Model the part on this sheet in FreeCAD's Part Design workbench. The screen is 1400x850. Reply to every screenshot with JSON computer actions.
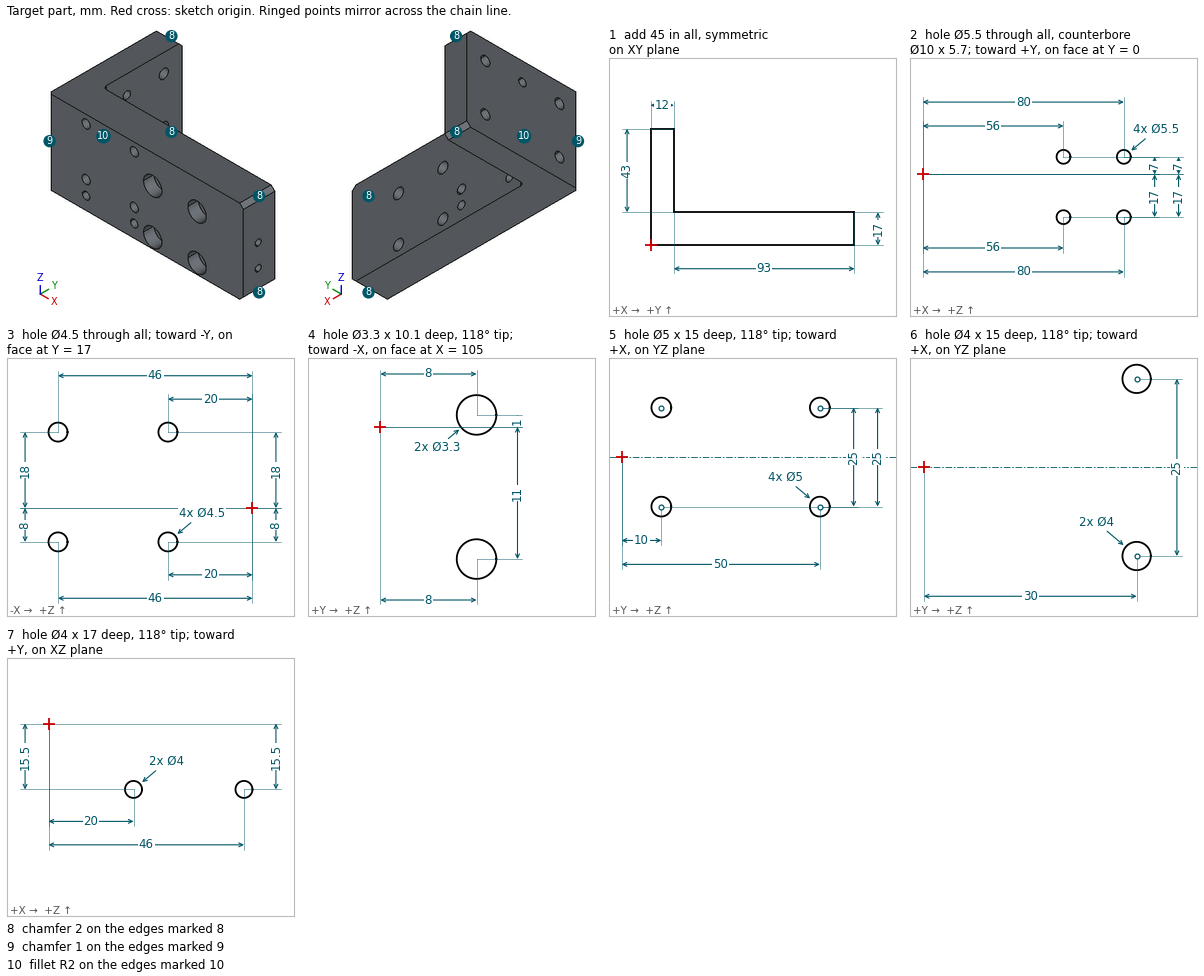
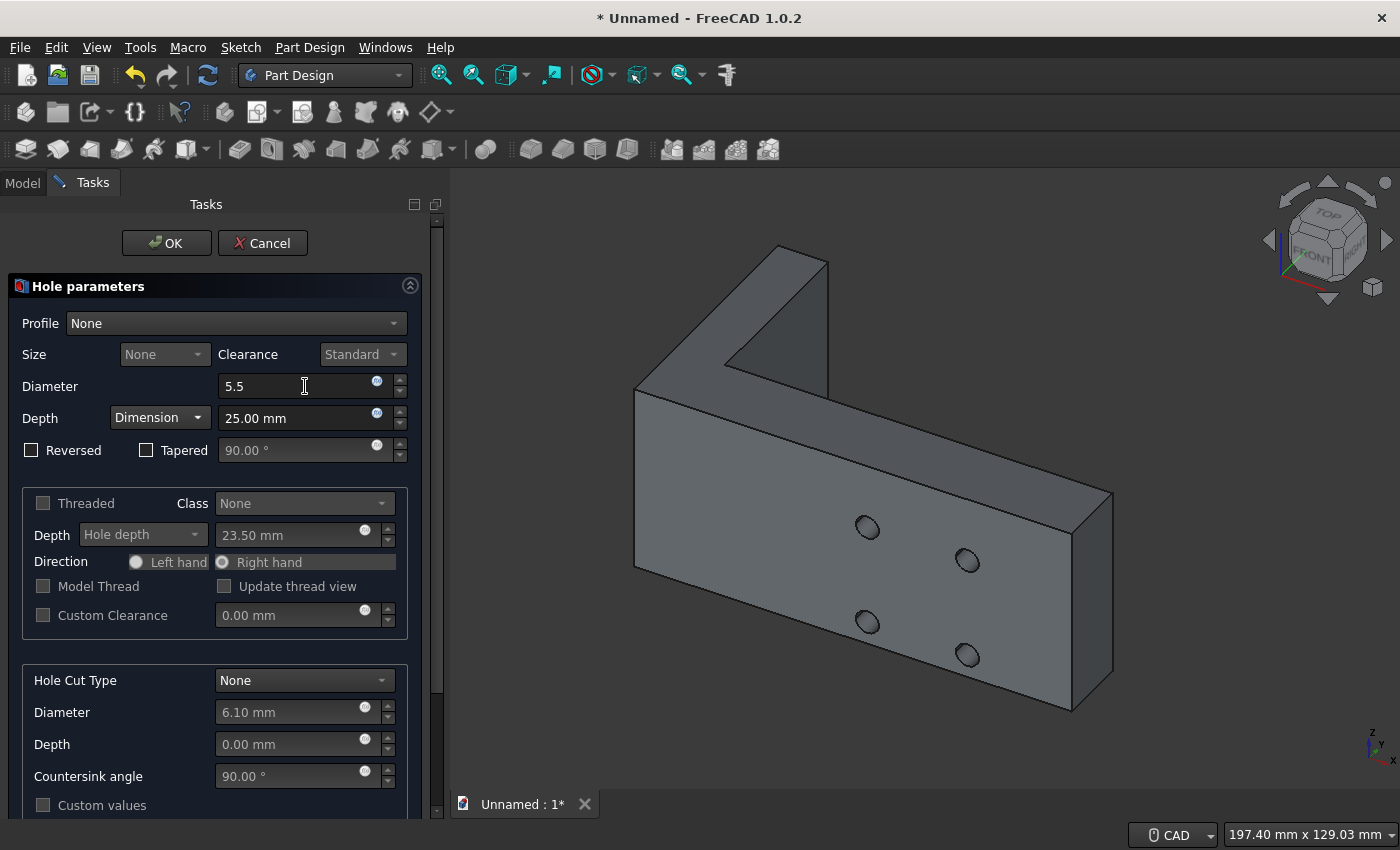
{"action": "left_click", "coordinate": [161, 418]}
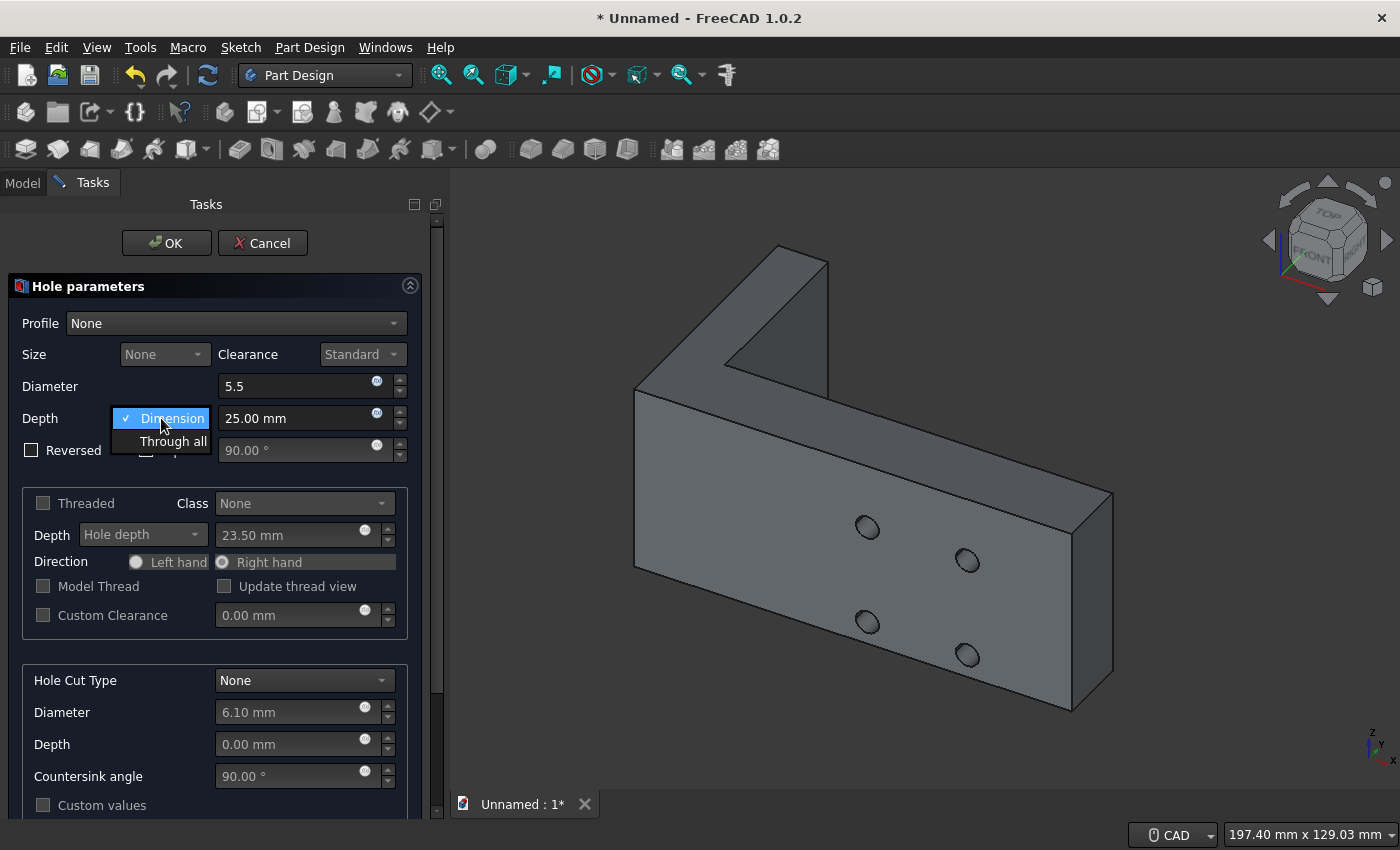
{"action": "left_click", "coordinate": [160, 442]}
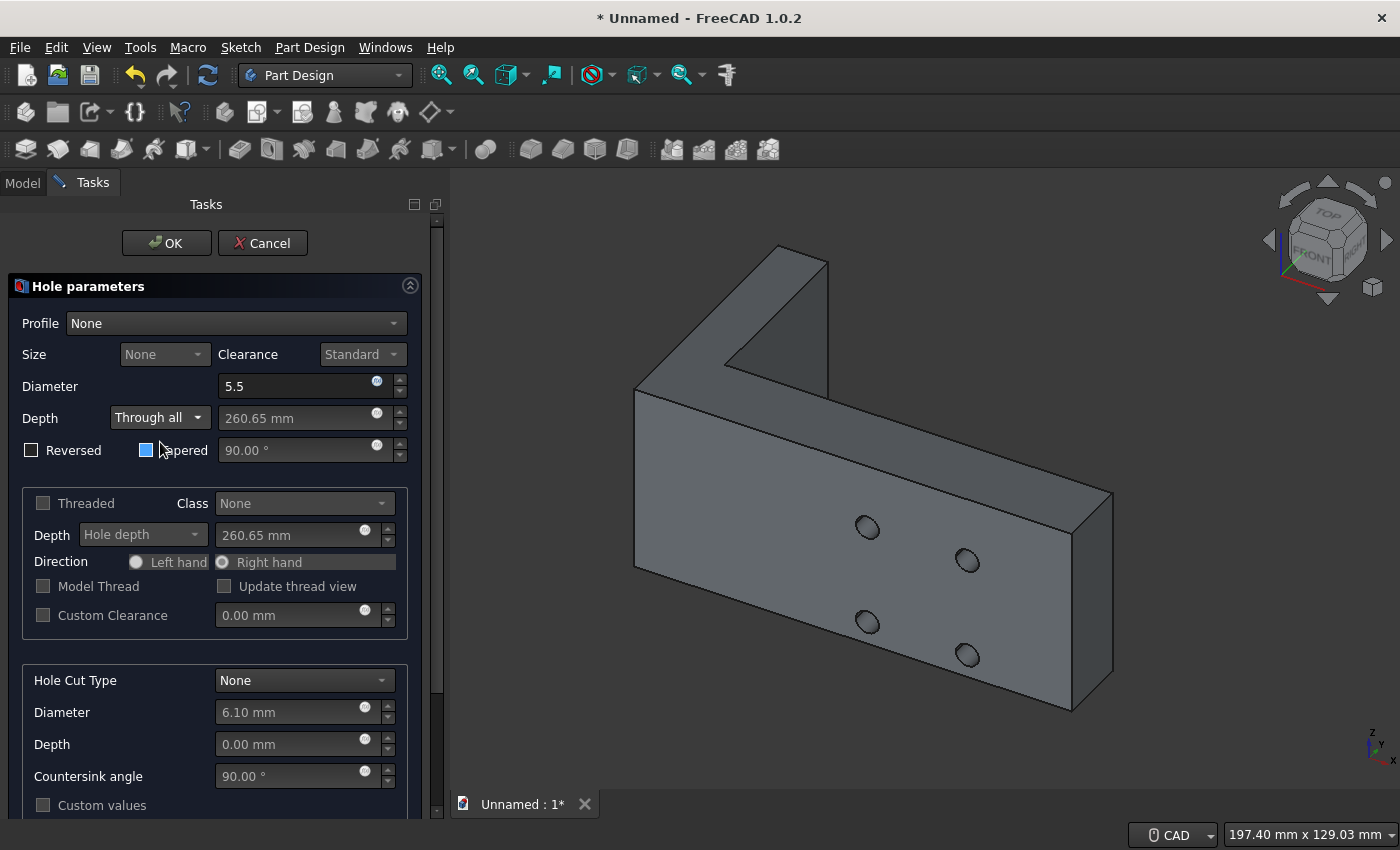
{"action": "left_click", "coordinate": [306, 680]}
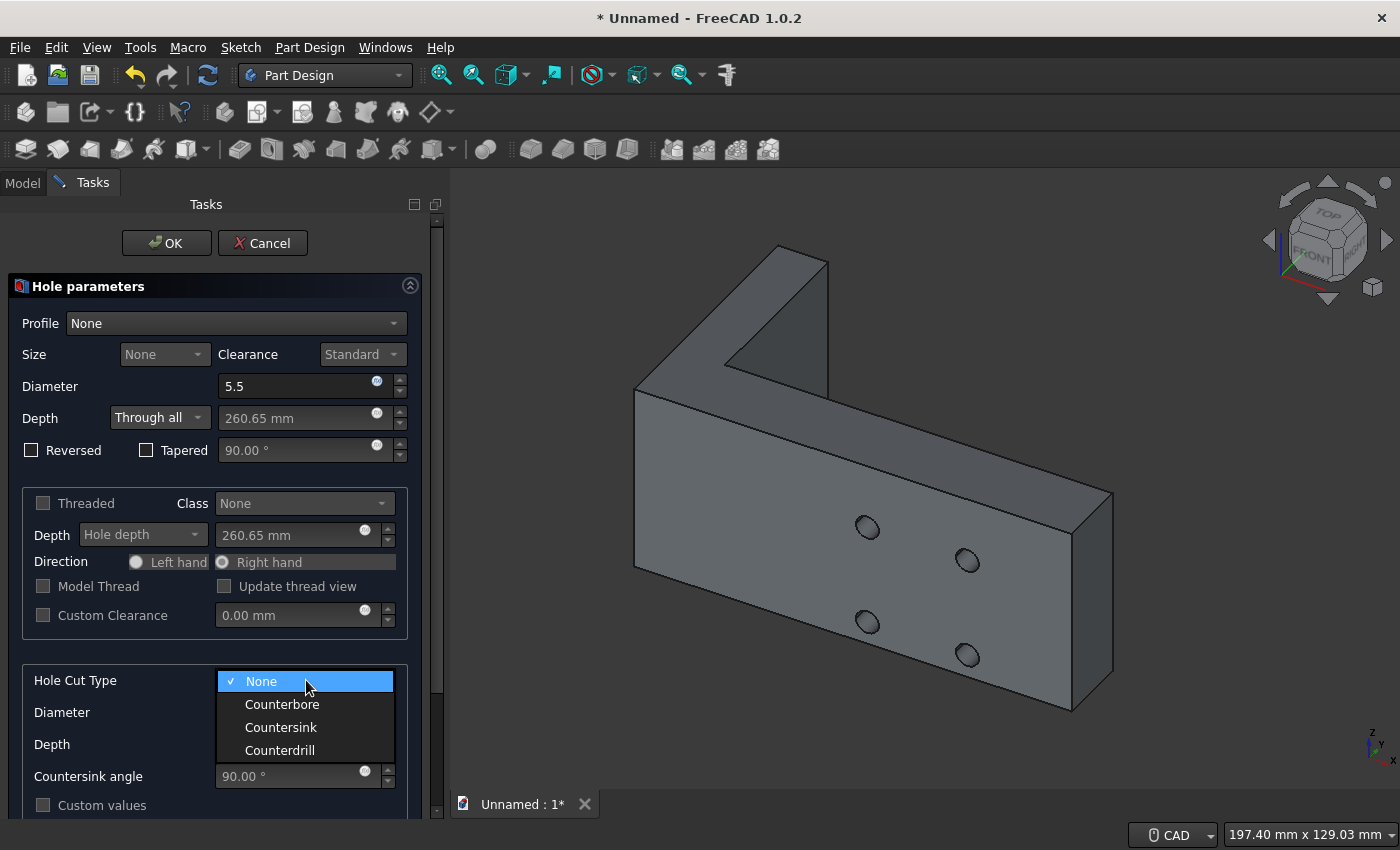
{"action": "left_click", "coordinate": [304, 704]}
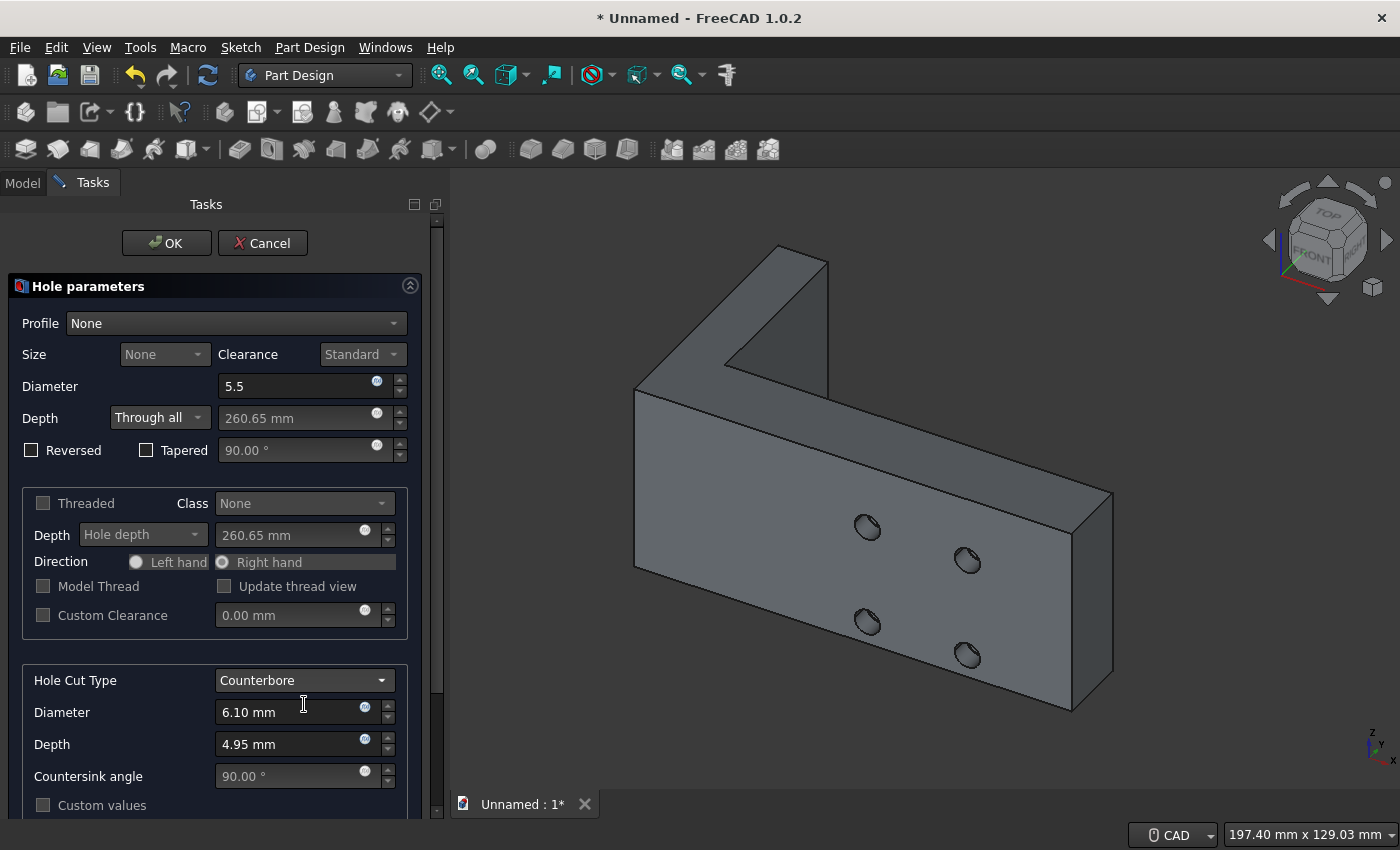
{"action": "triple_click", "coordinate": [298, 712]}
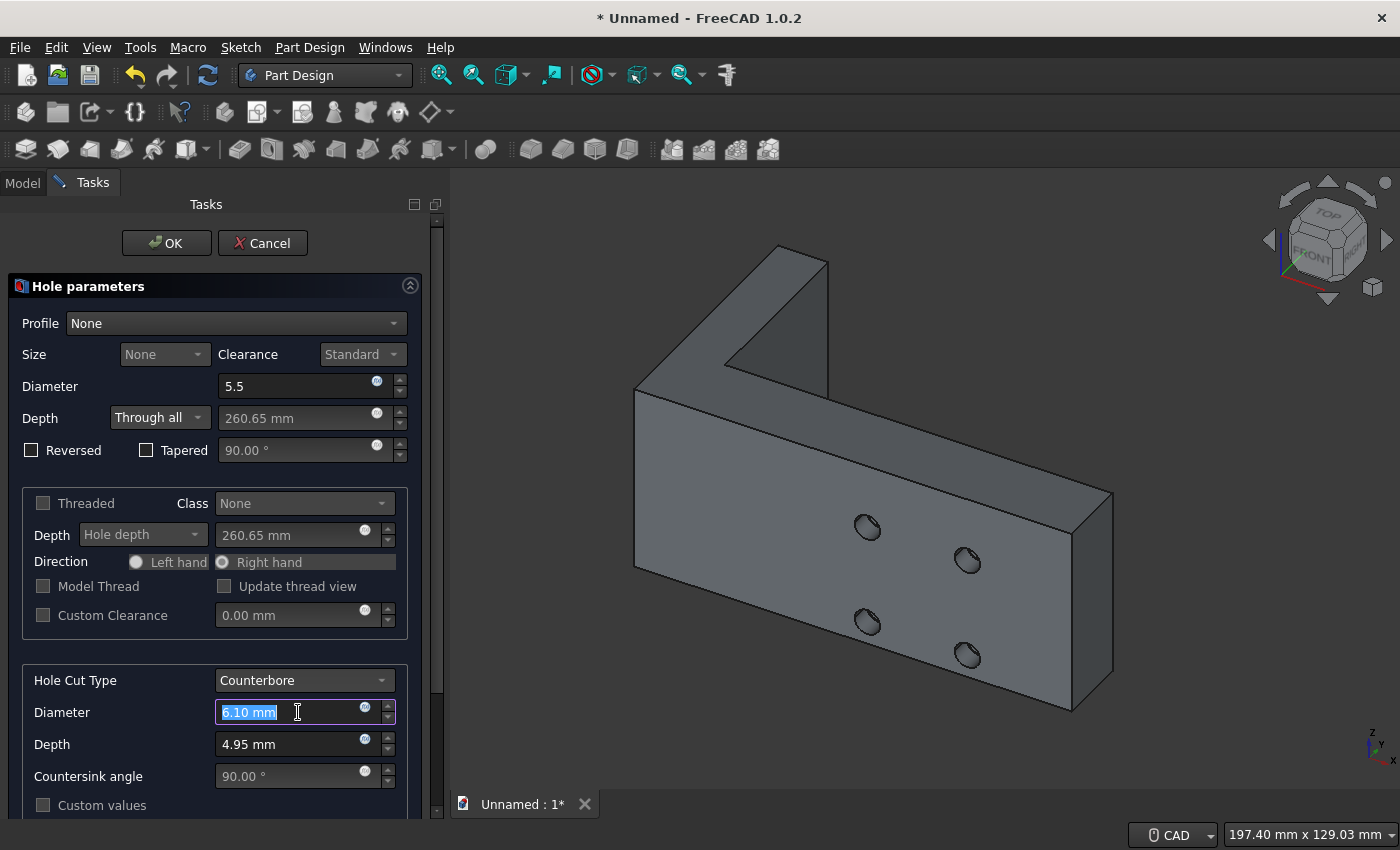
{"action": "type", "text": "10"}
{"action": "key", "text": "Tab"}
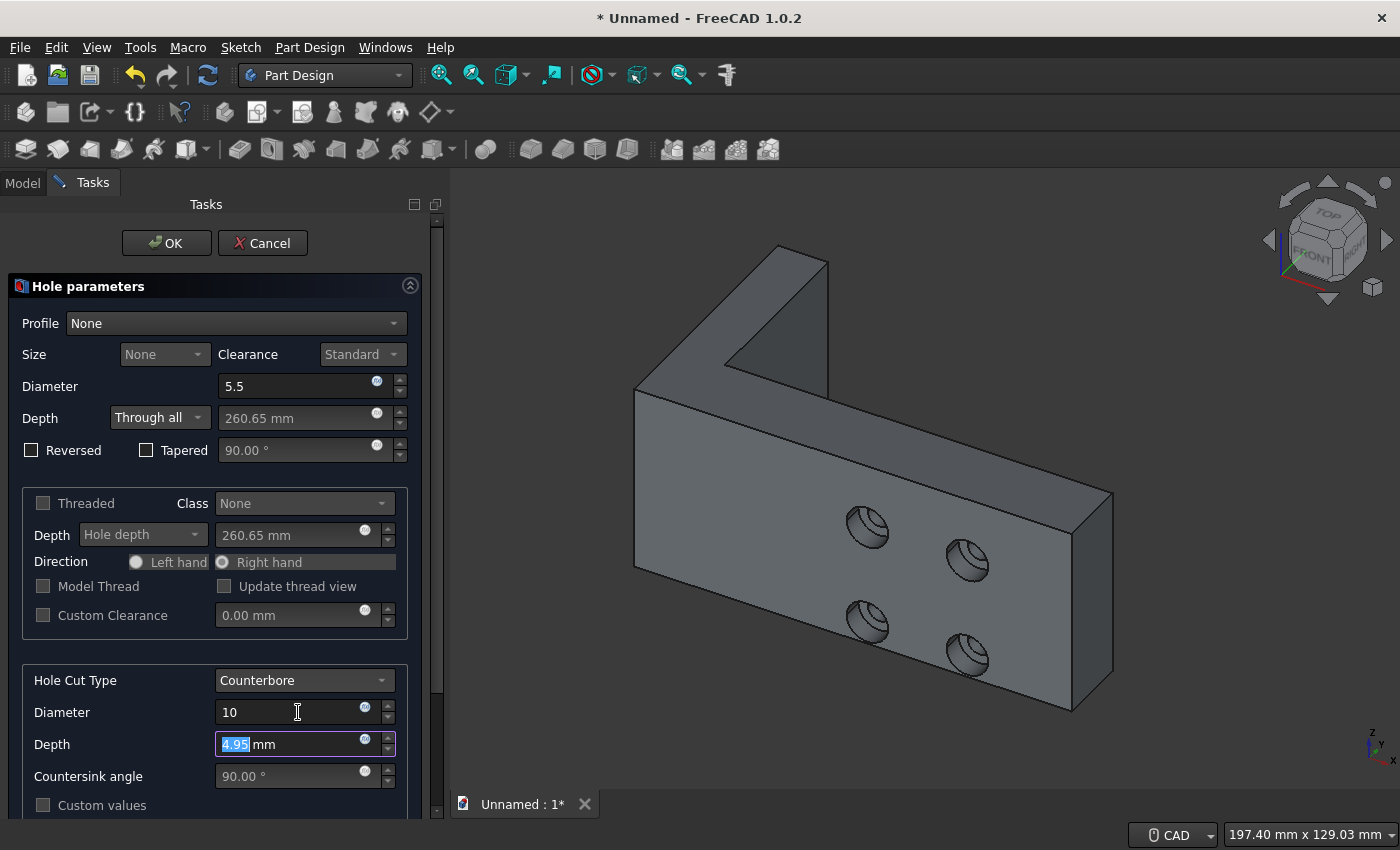
{"action": "type", "text": "5.7"}
{"action": "key", "text": "Tab"}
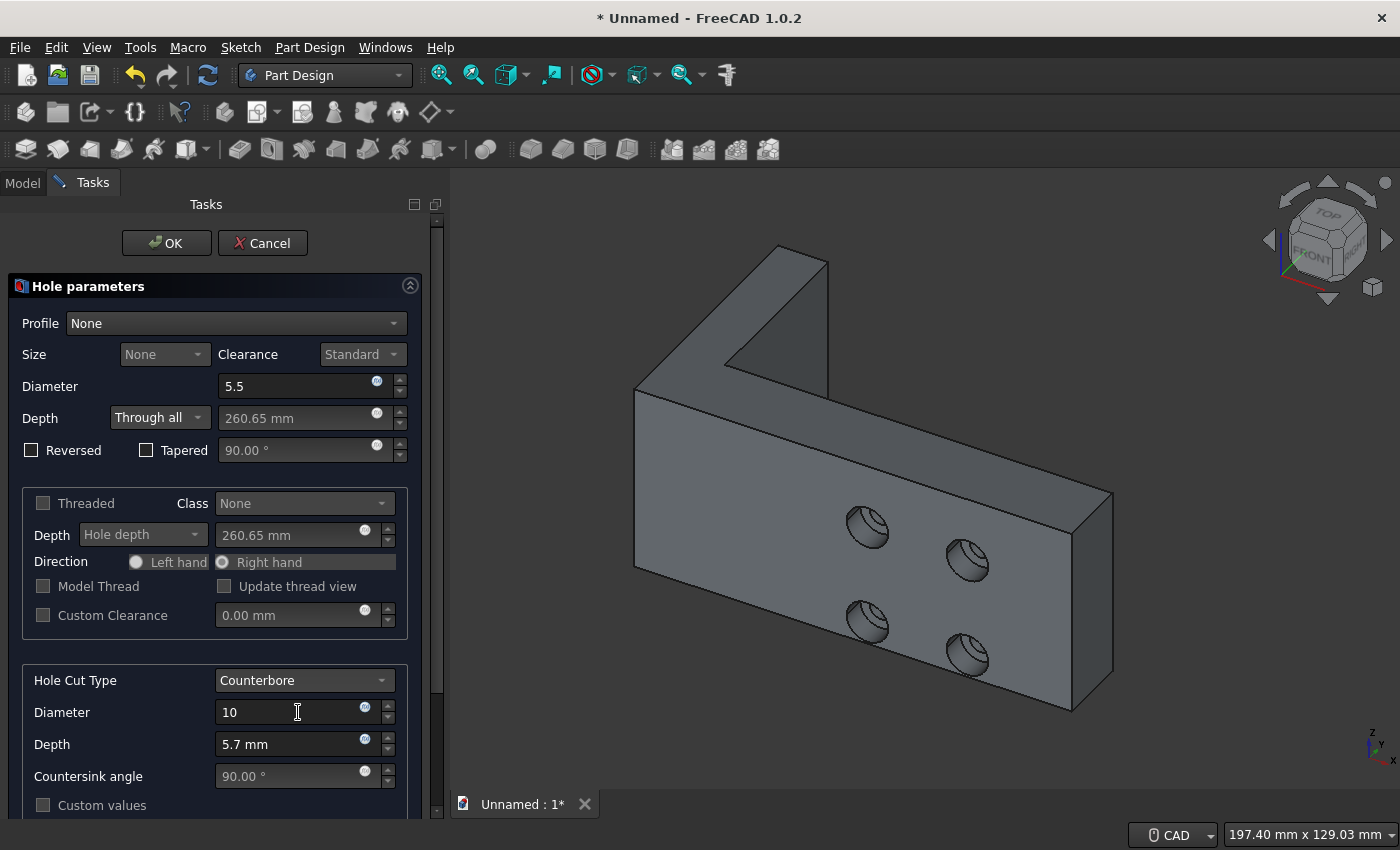
{"action": "left_click", "coordinate": [167, 243]}